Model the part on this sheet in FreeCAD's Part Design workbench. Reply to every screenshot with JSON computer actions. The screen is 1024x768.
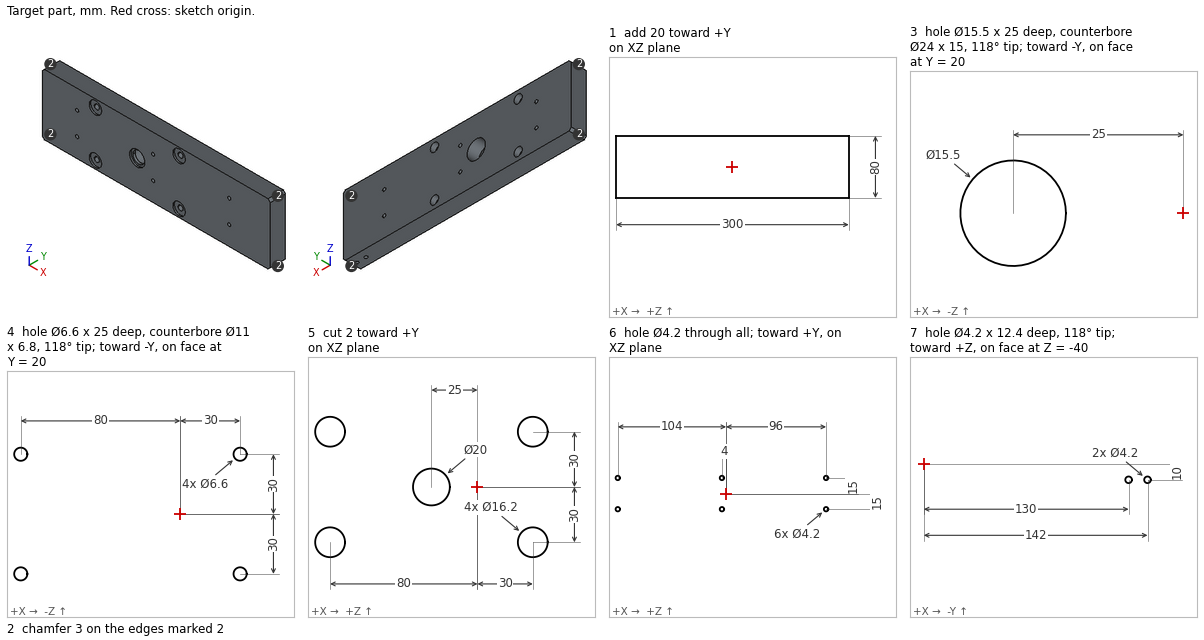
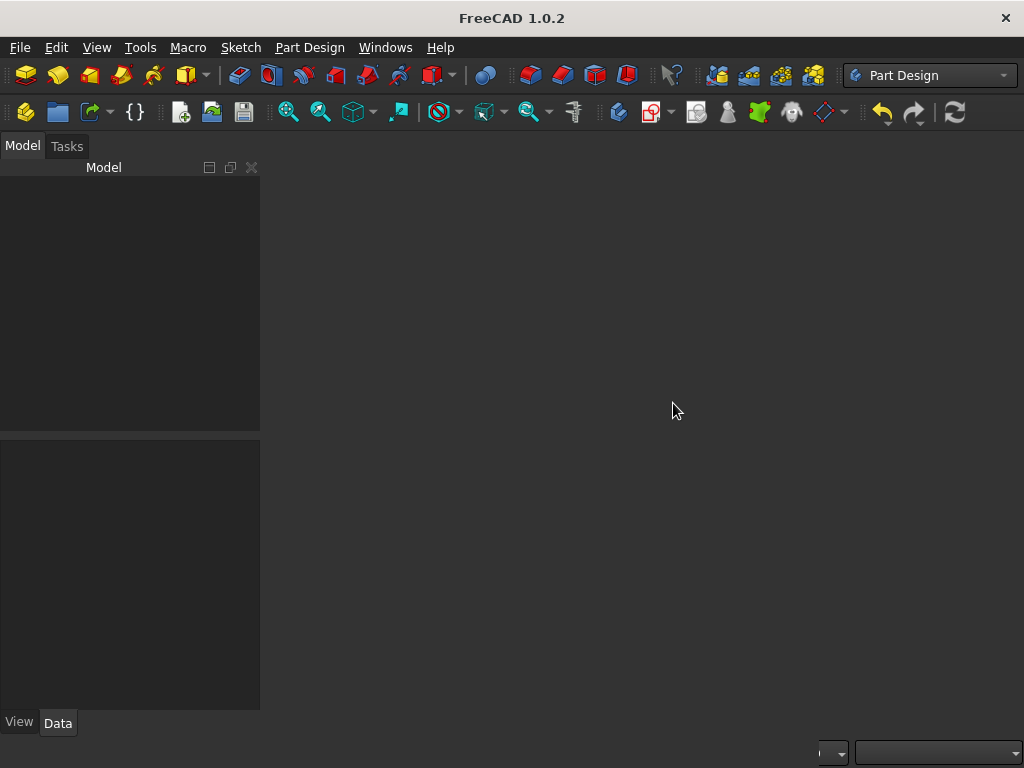
{"action": "left_click", "coordinate": [180, 112]}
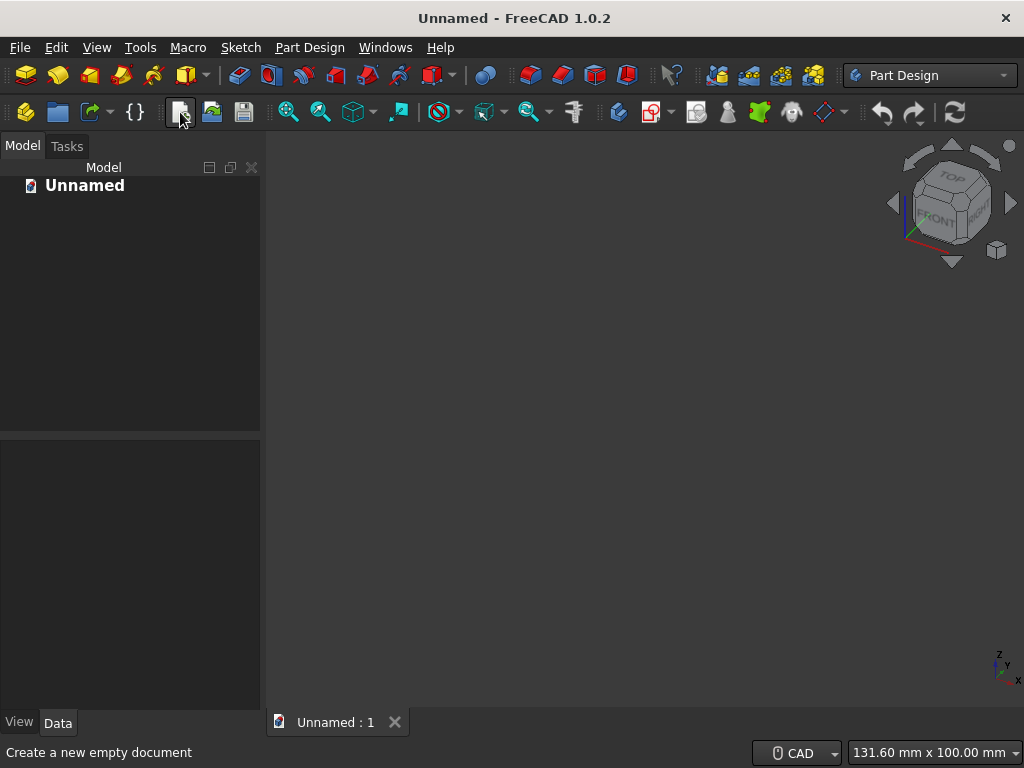
{"action": "left_click", "coordinate": [652, 112]}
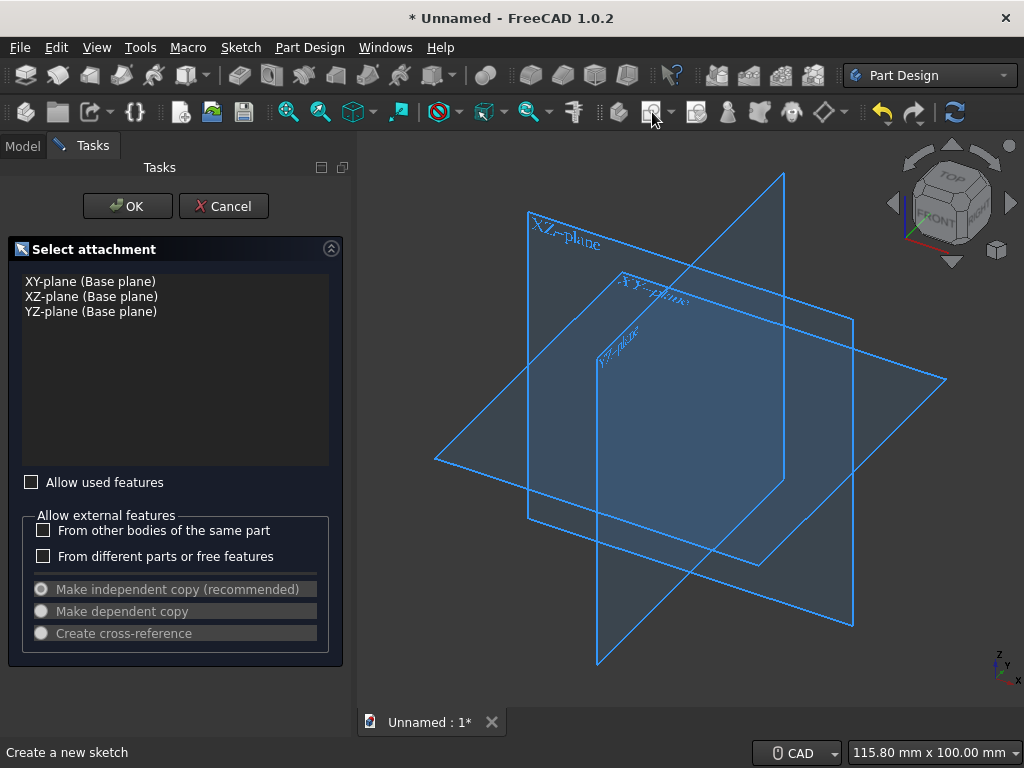
{"action": "left_click", "coordinate": [82, 296]}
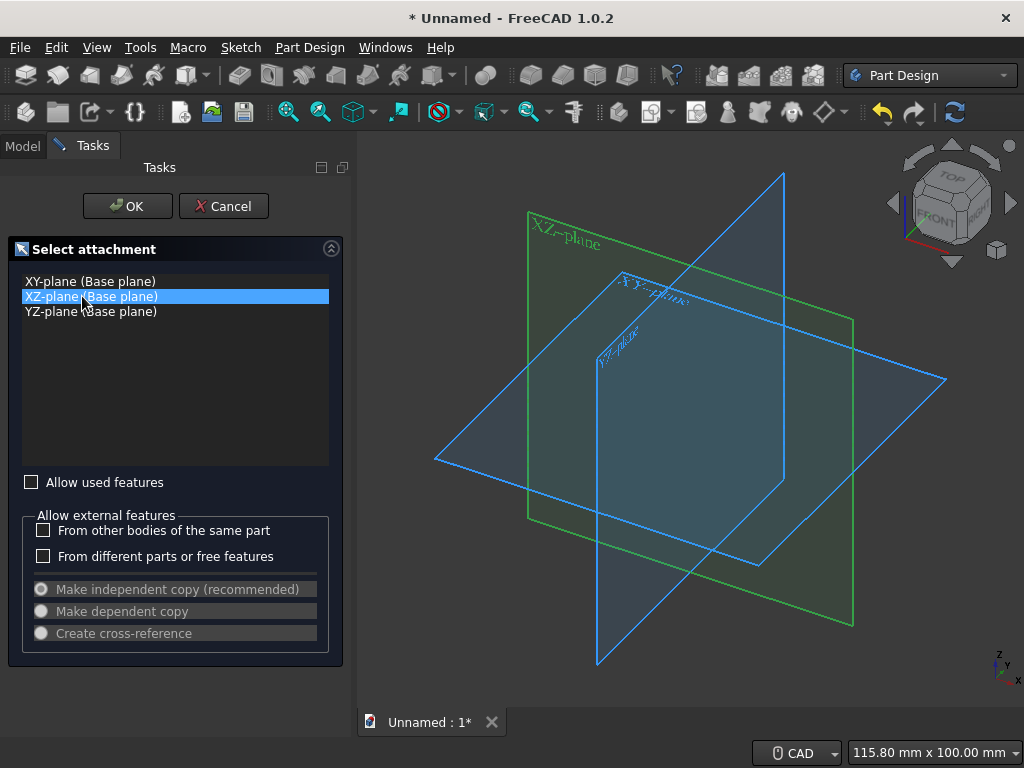
{"action": "left_click", "coordinate": [128, 206]}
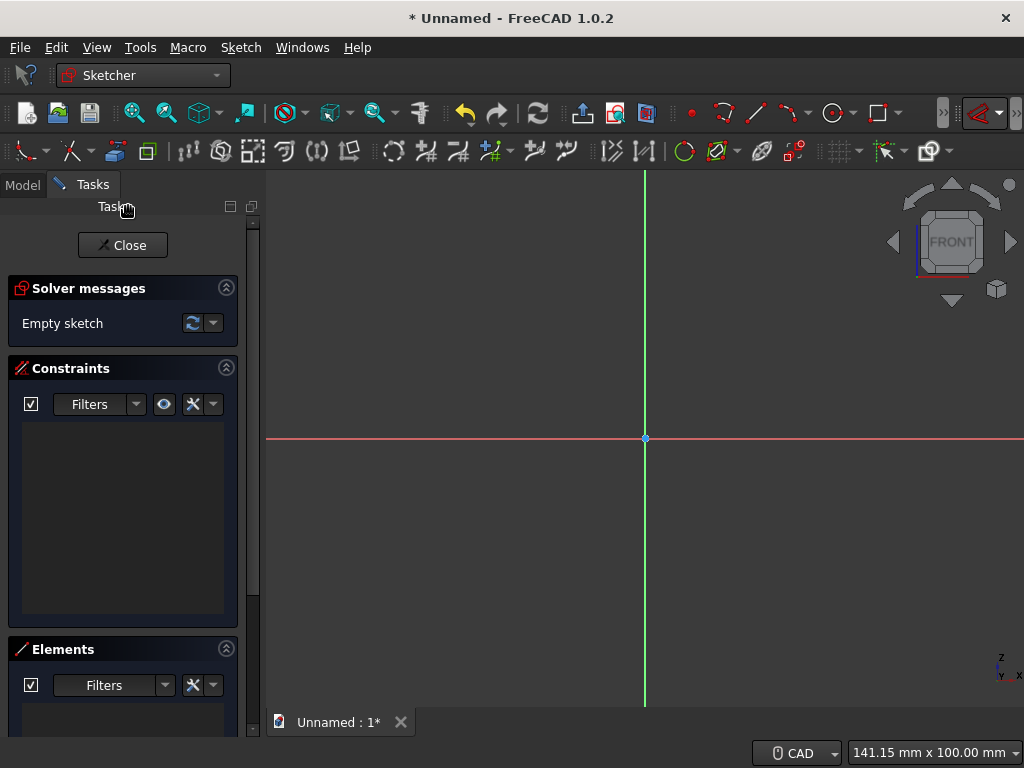
{"action": "scroll", "coordinate": [554, 438], "scroll_direction": "down", "scroll_amount": 7}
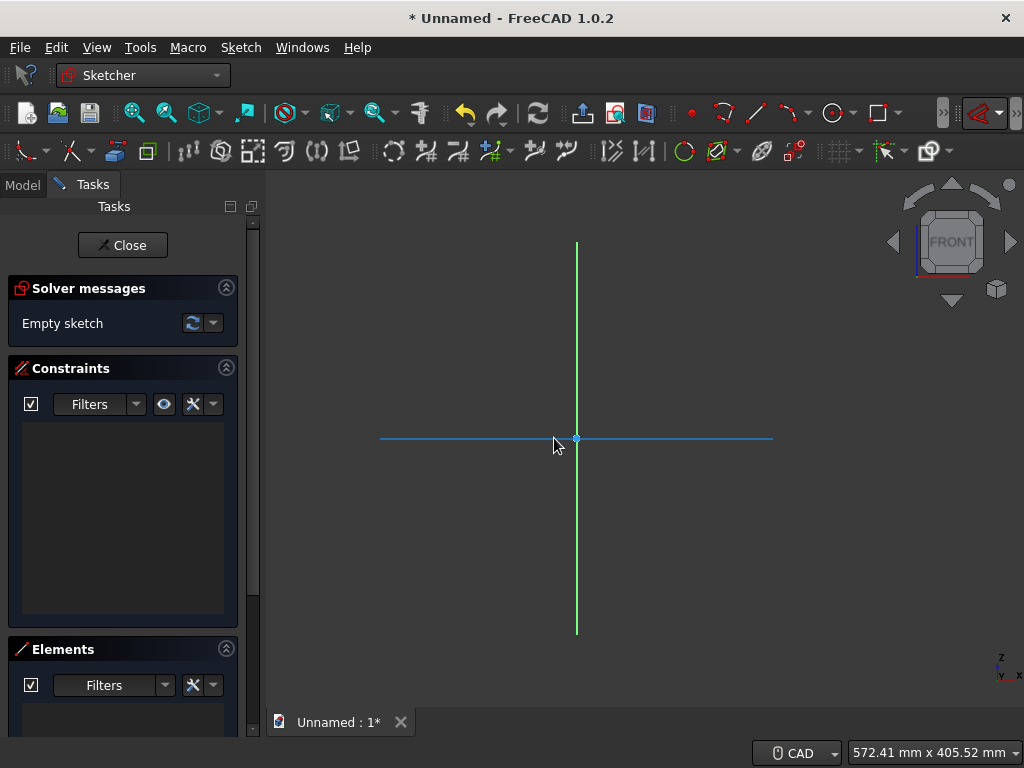
{"action": "key", "text": "g v"}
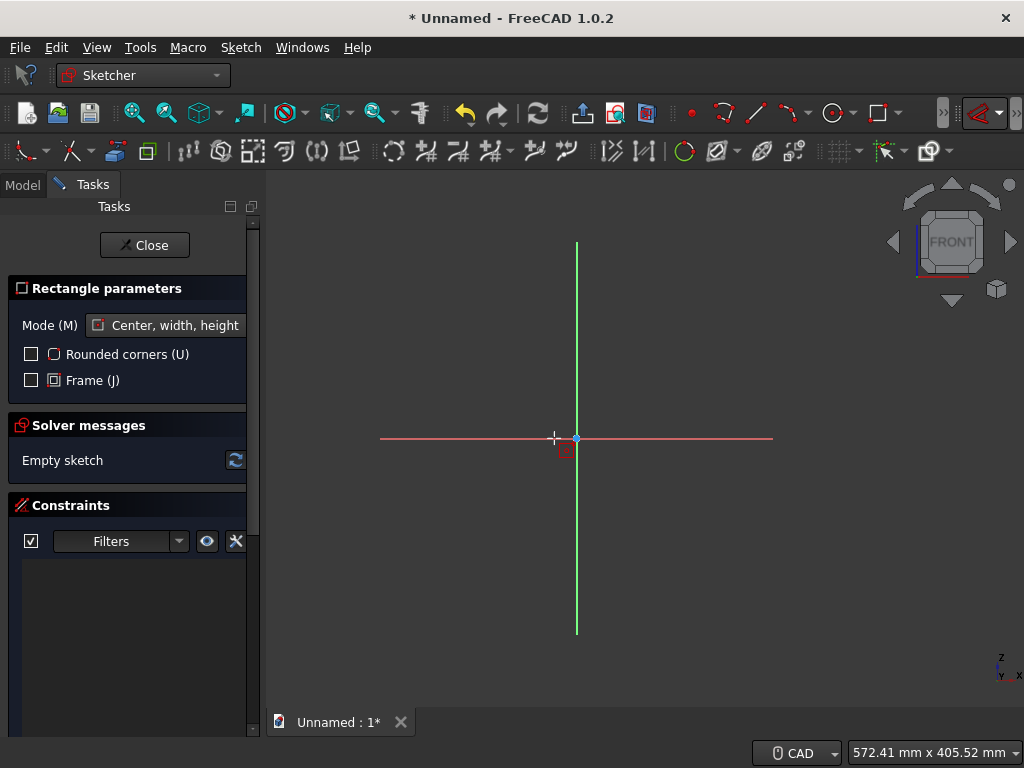
{"action": "left_click", "coordinate": [577, 438]}
{"action": "mouse_move", "coordinate": [775, 386]}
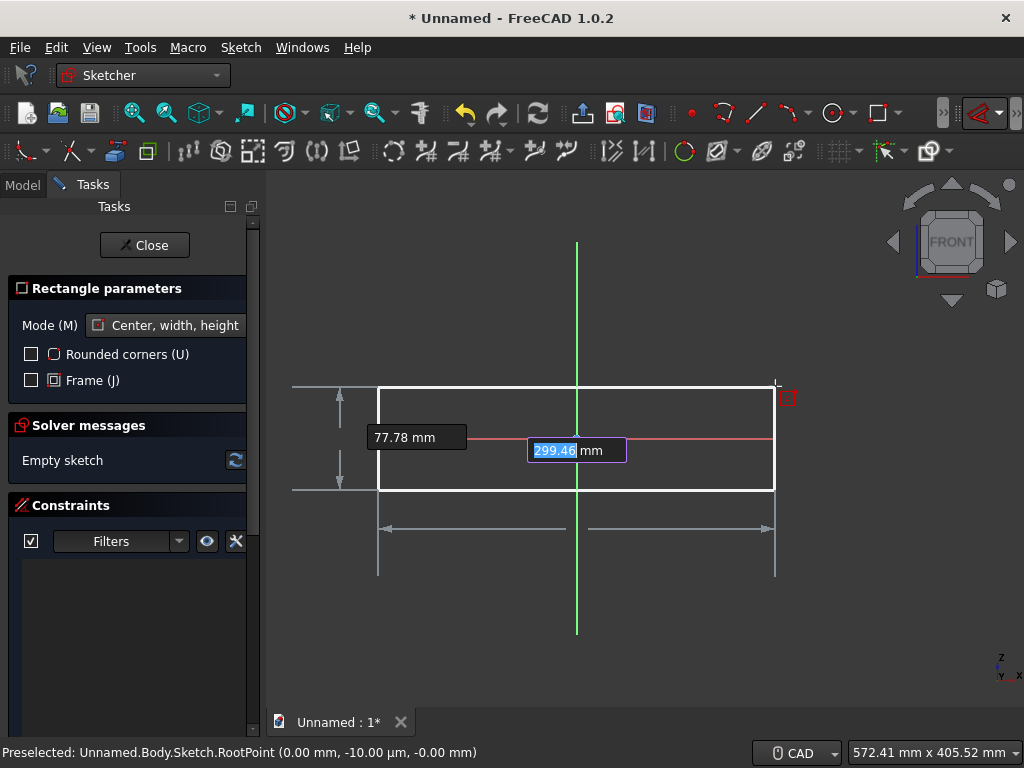
{"action": "type", "text": "300"}
{"action": "key", "text": "Tab"}
{"action": "type", "text": "80"}
{"action": "key", "text": "Return"}
{"action": "key", "text": "Escape"}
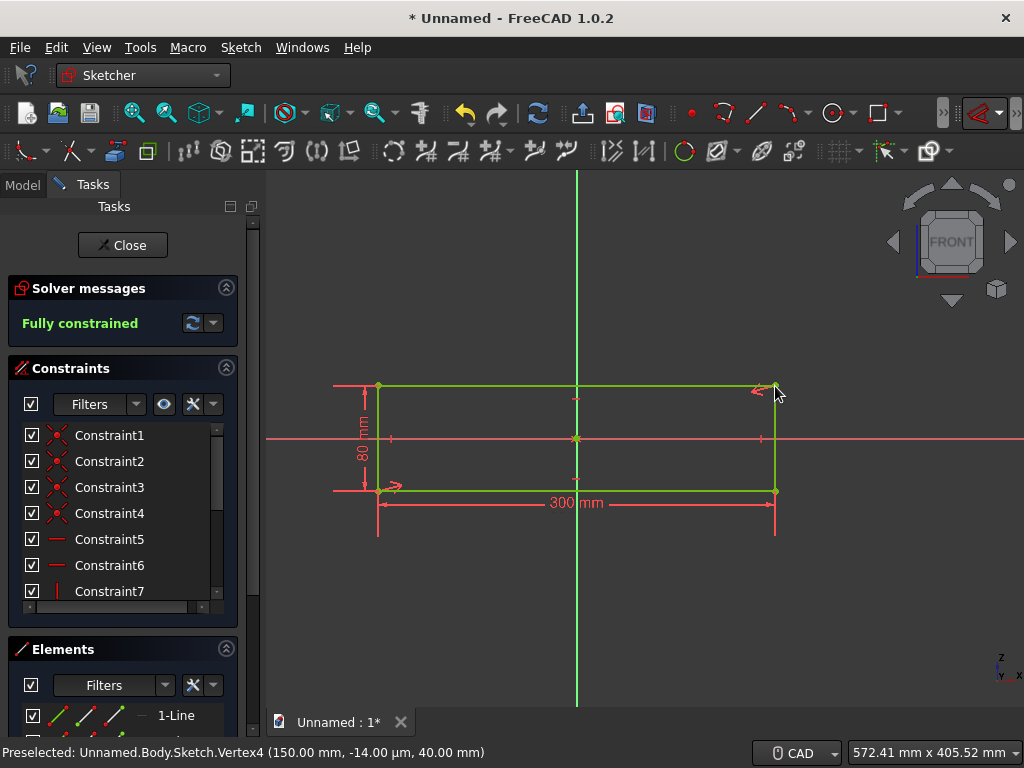
{"action": "left_click", "coordinate": [123, 245]}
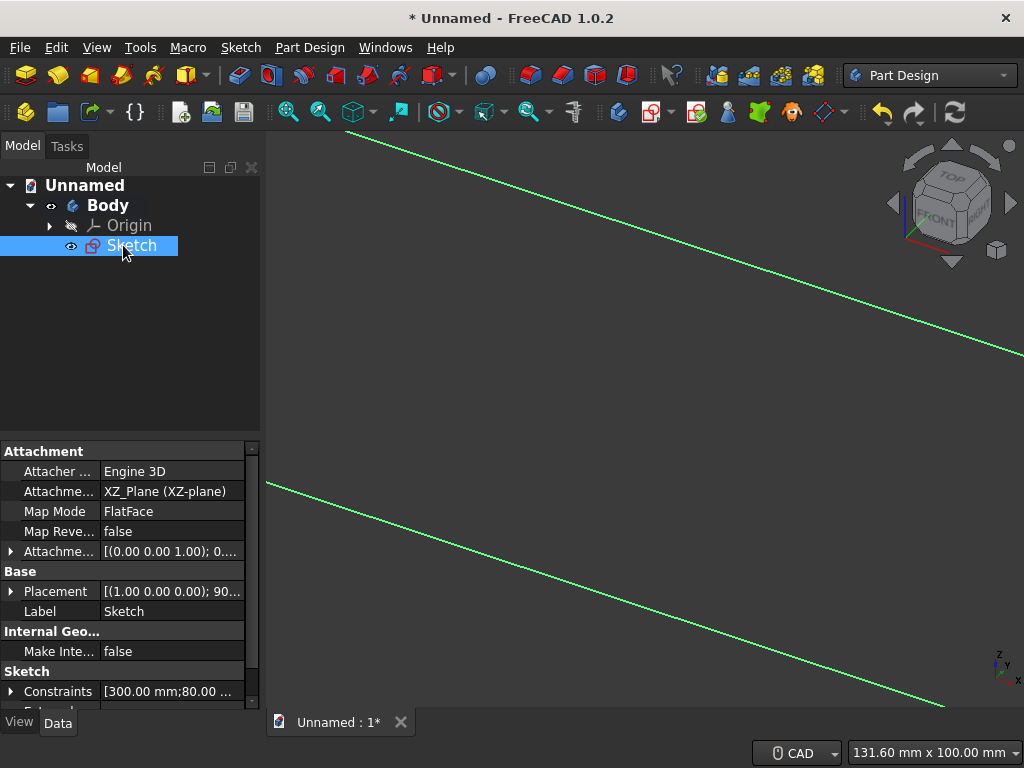
{"action": "left_click", "coordinate": [26, 76]}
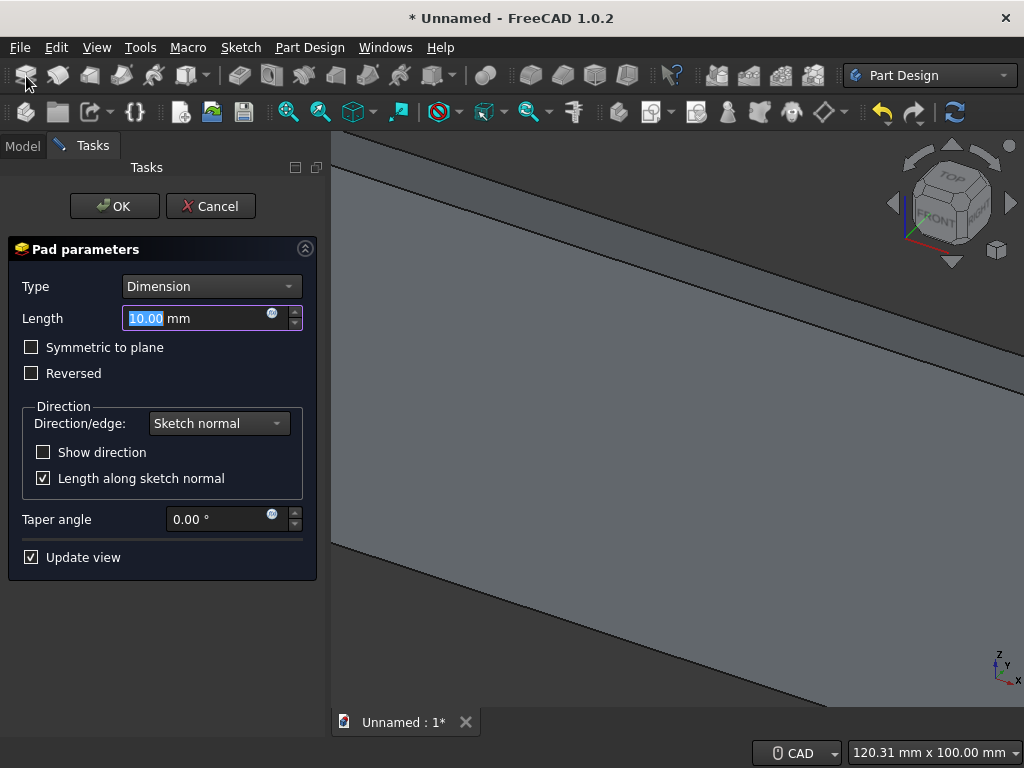
{"action": "type", "text": "20"}
{"action": "key", "text": "Tab"}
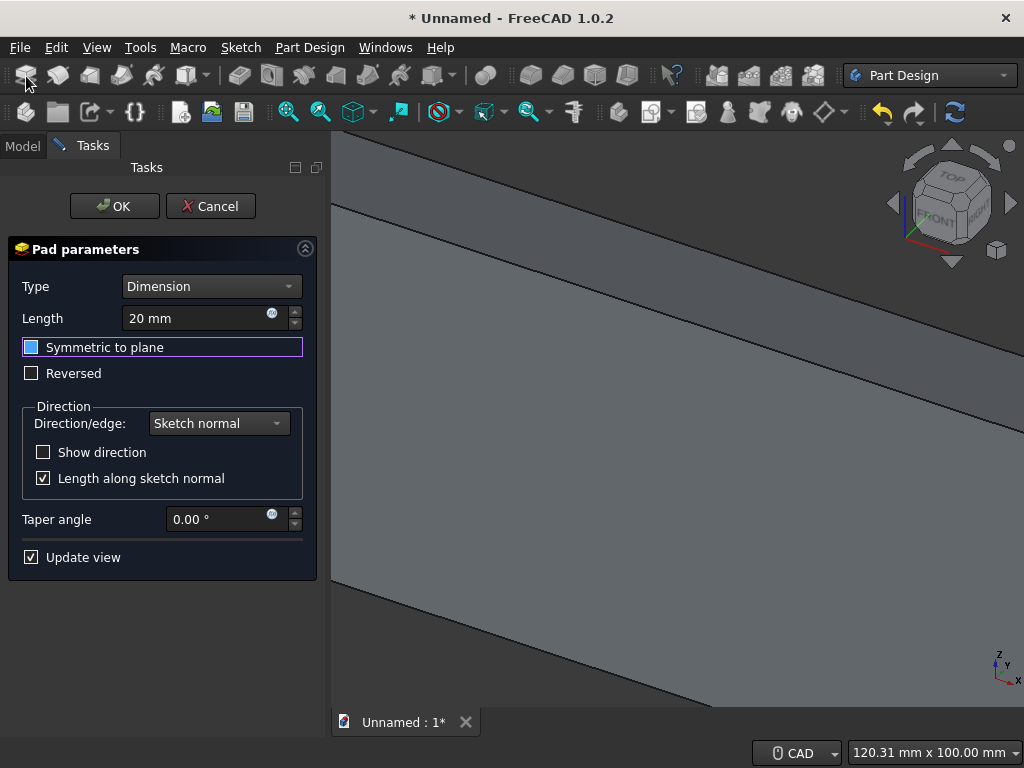
{"action": "left_click", "coordinate": [30, 373]}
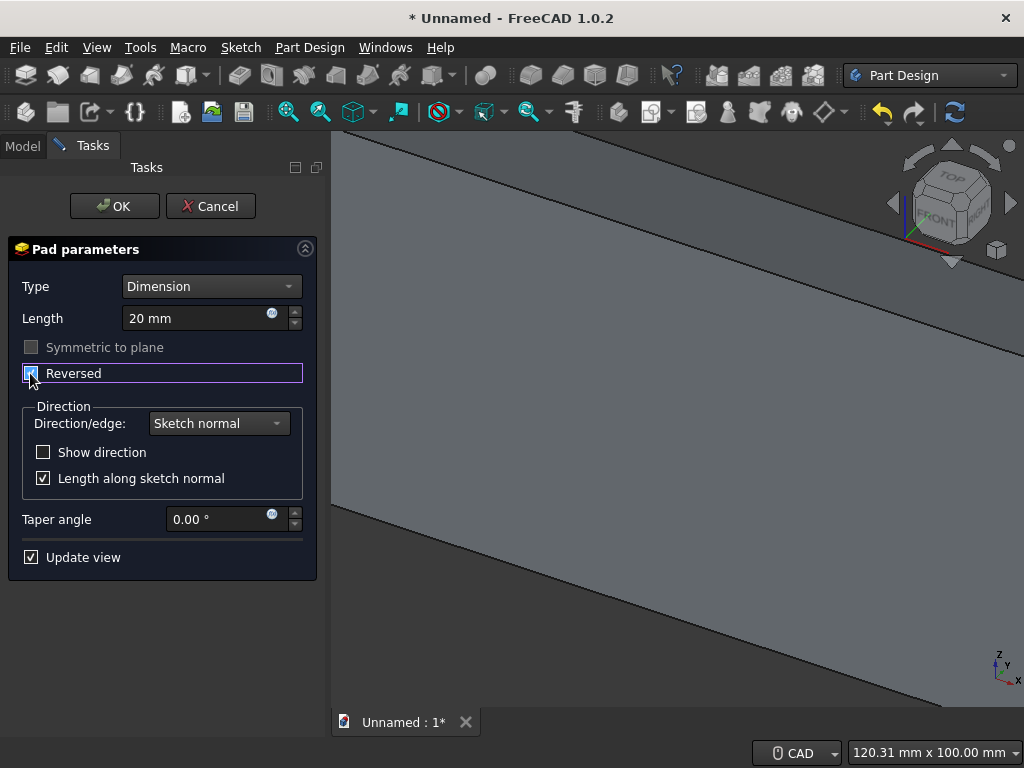
{"action": "left_click", "coordinate": [115, 206]}